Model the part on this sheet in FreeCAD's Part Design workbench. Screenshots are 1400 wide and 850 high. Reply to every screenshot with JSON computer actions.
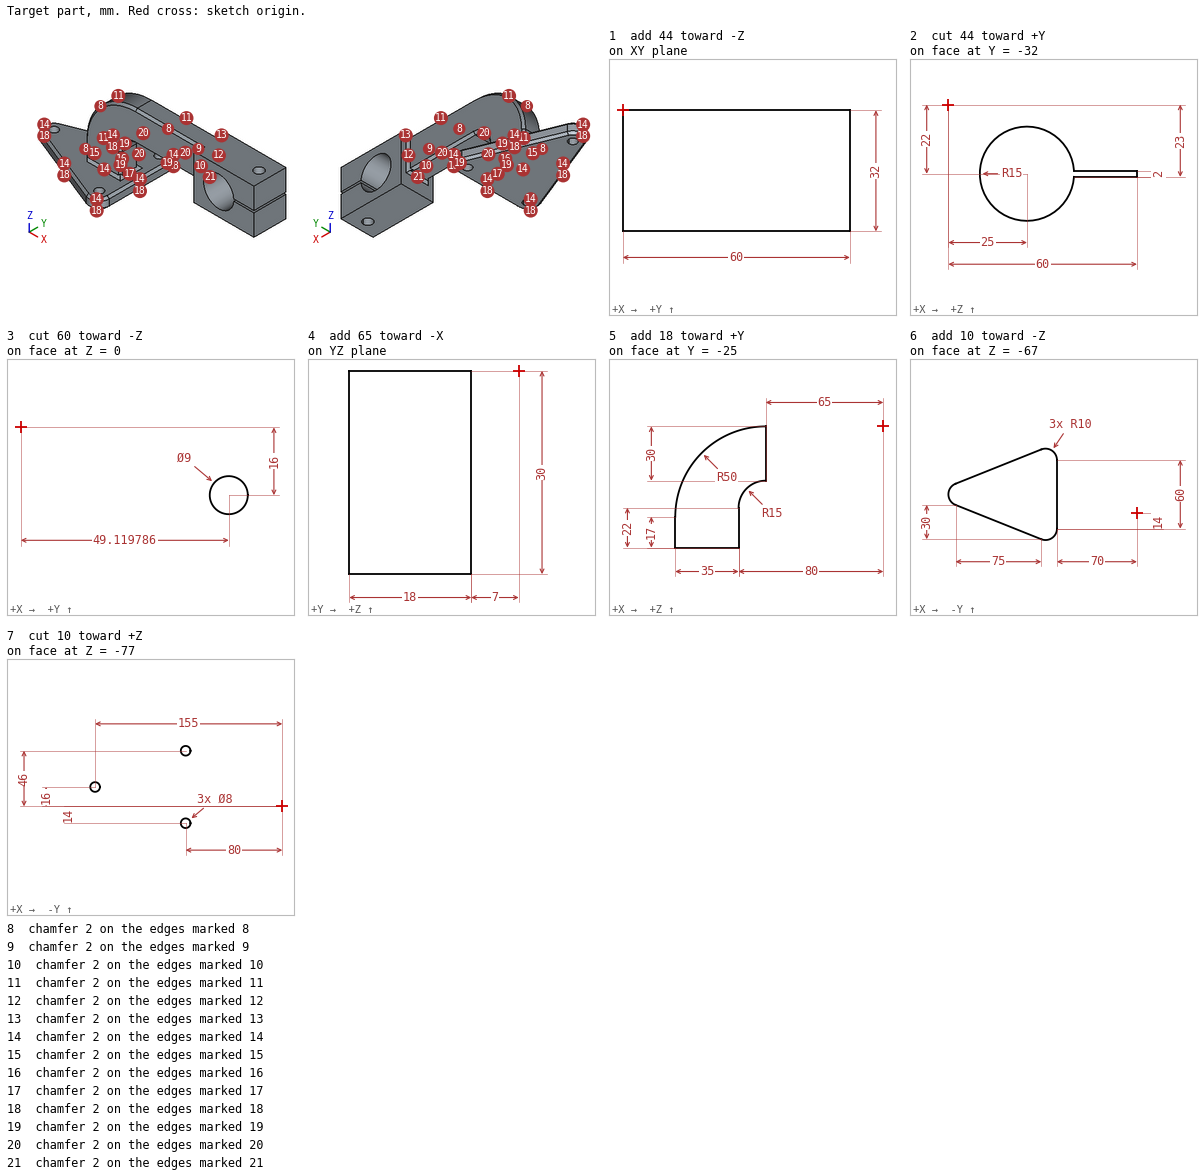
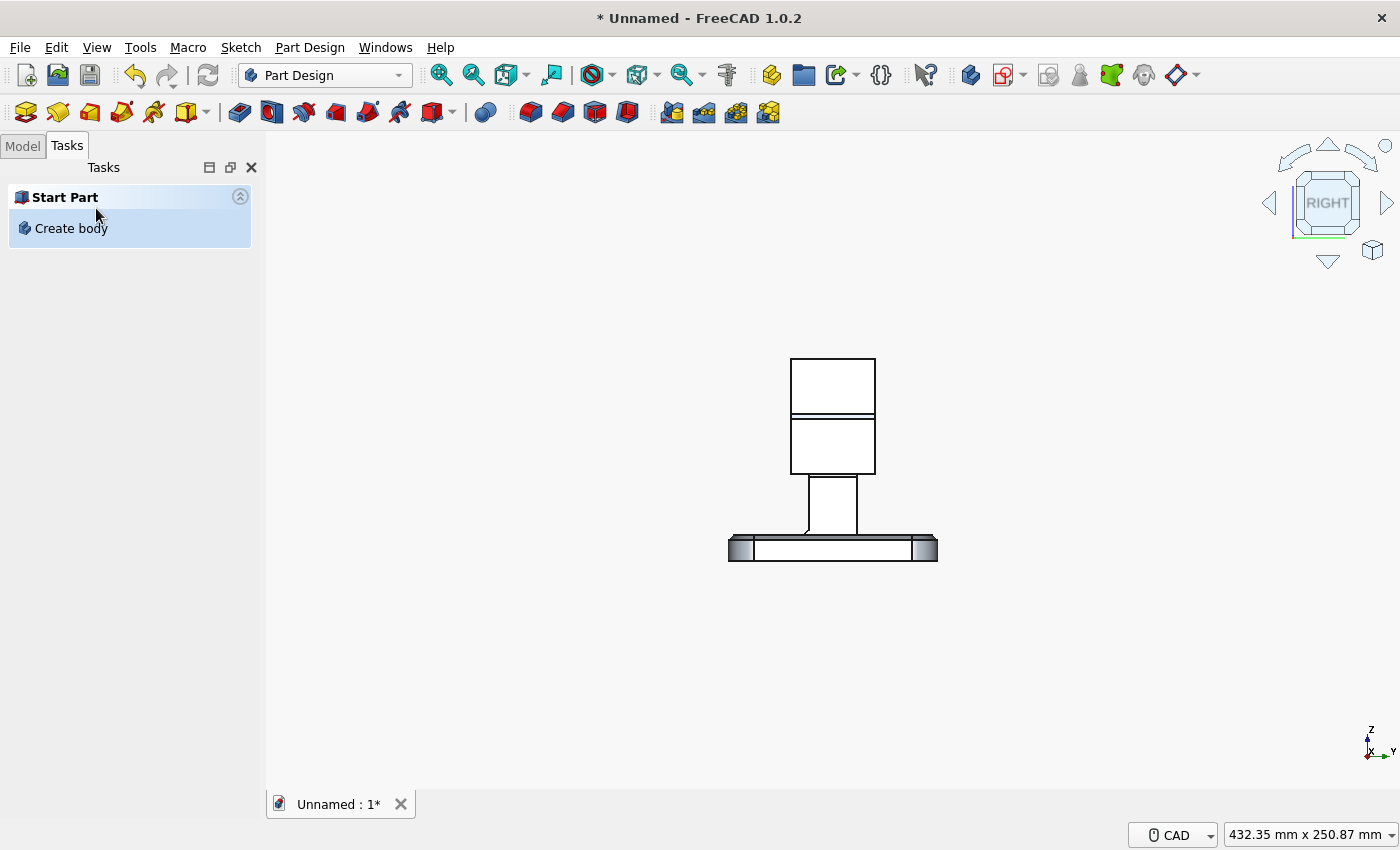
{"action": "key", "text": "5"}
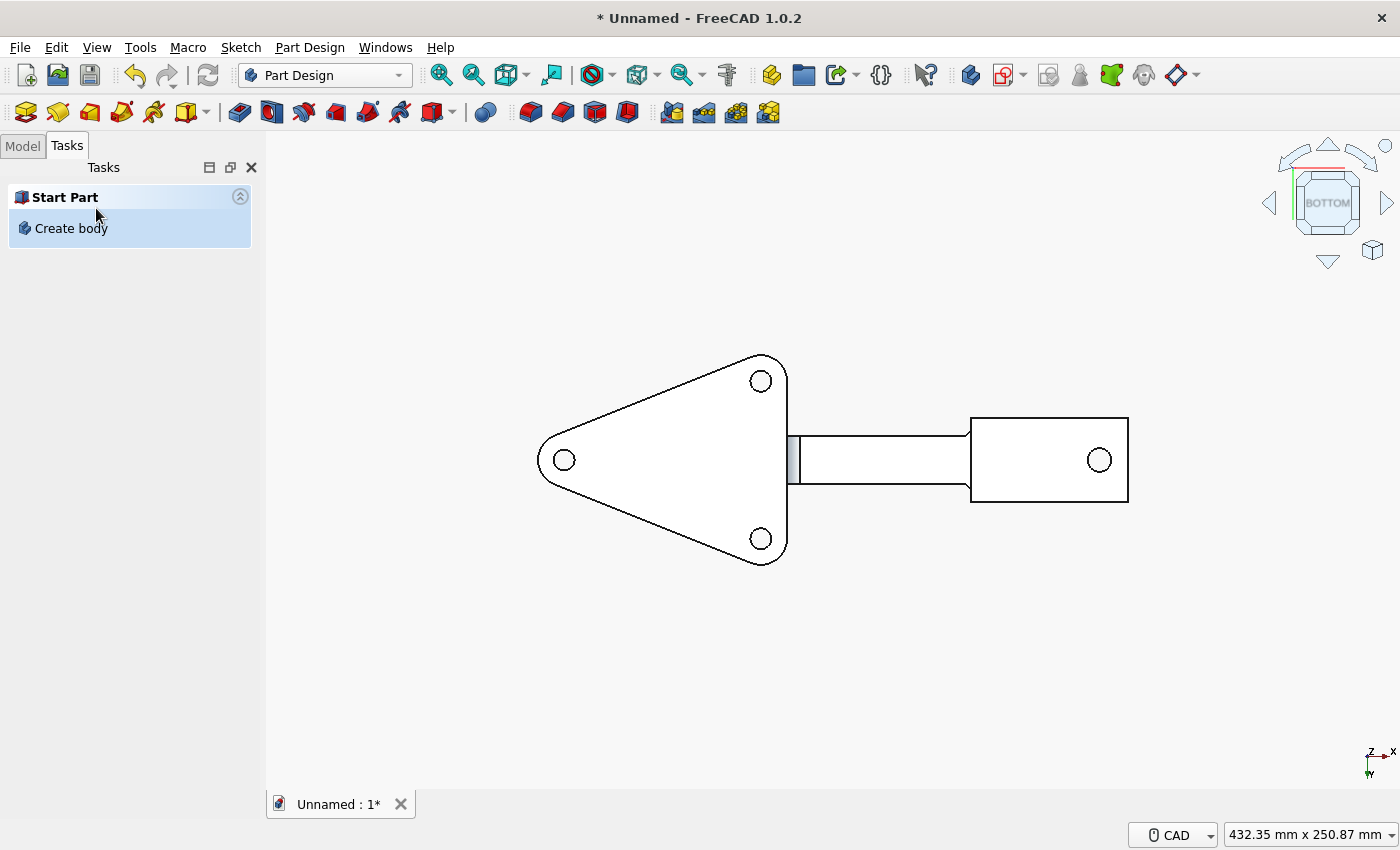
{"action": "key", "text": "4"}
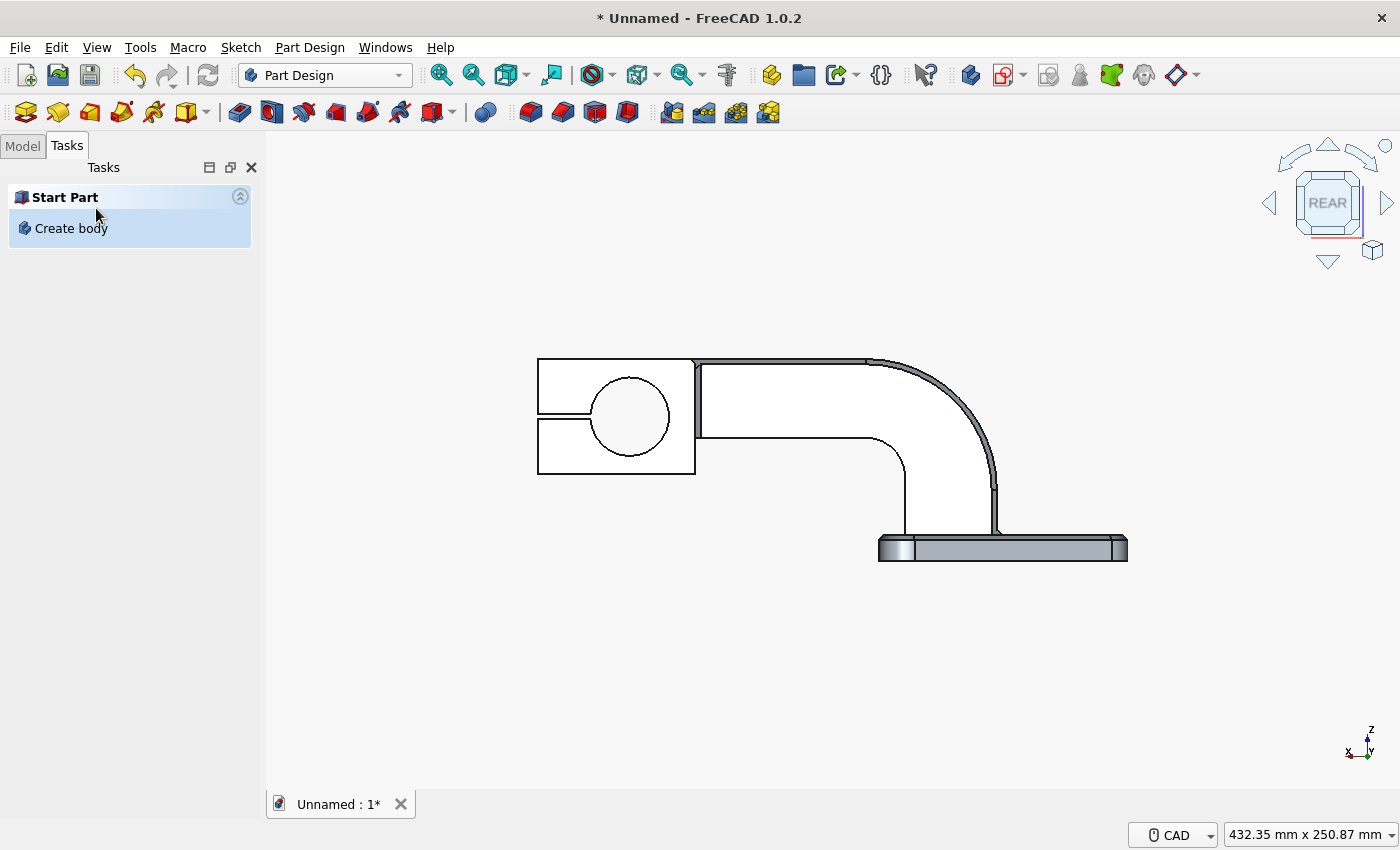
{"action": "key", "text": "6"}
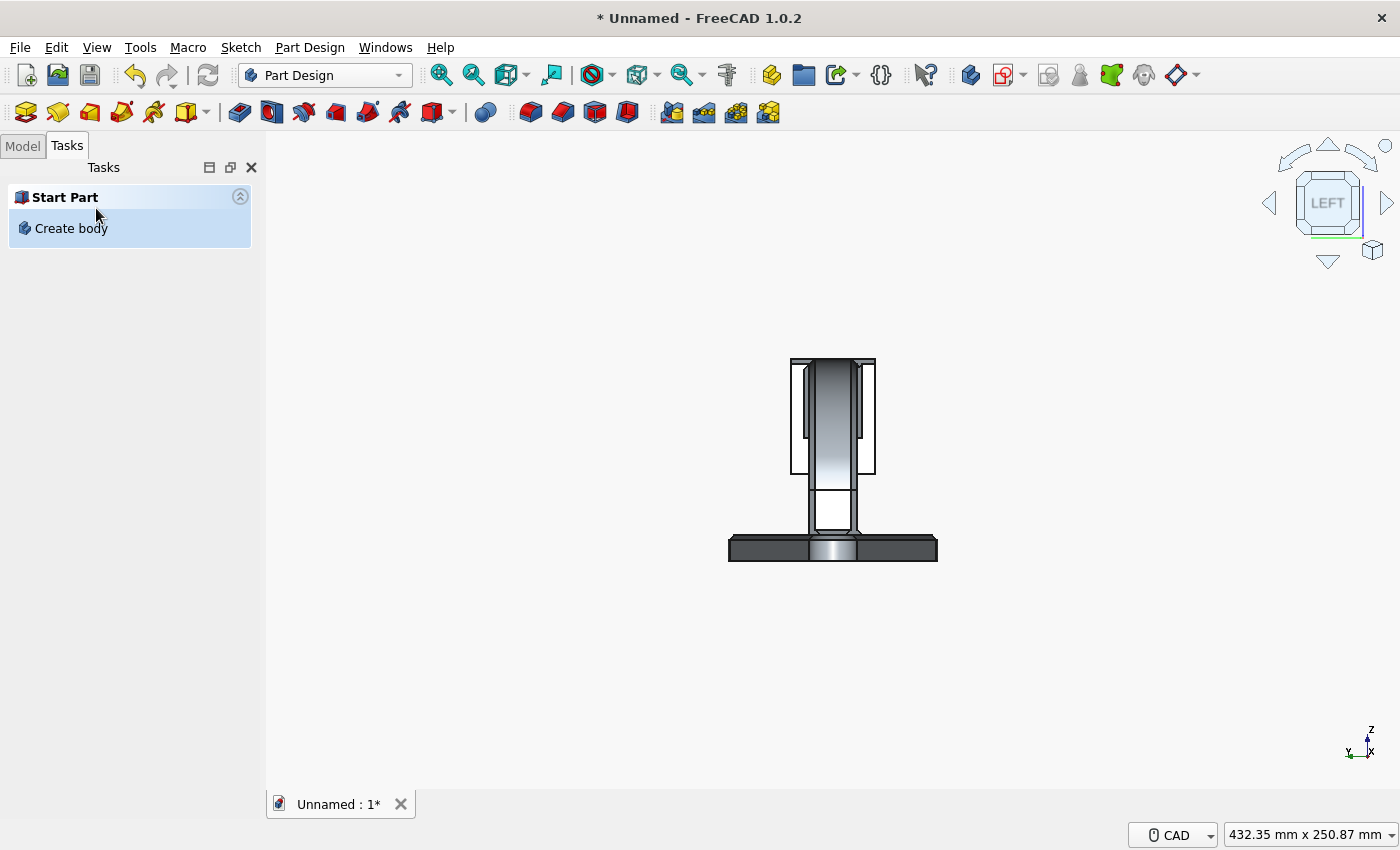
{"action": "left_click", "coordinate": [442, 76]}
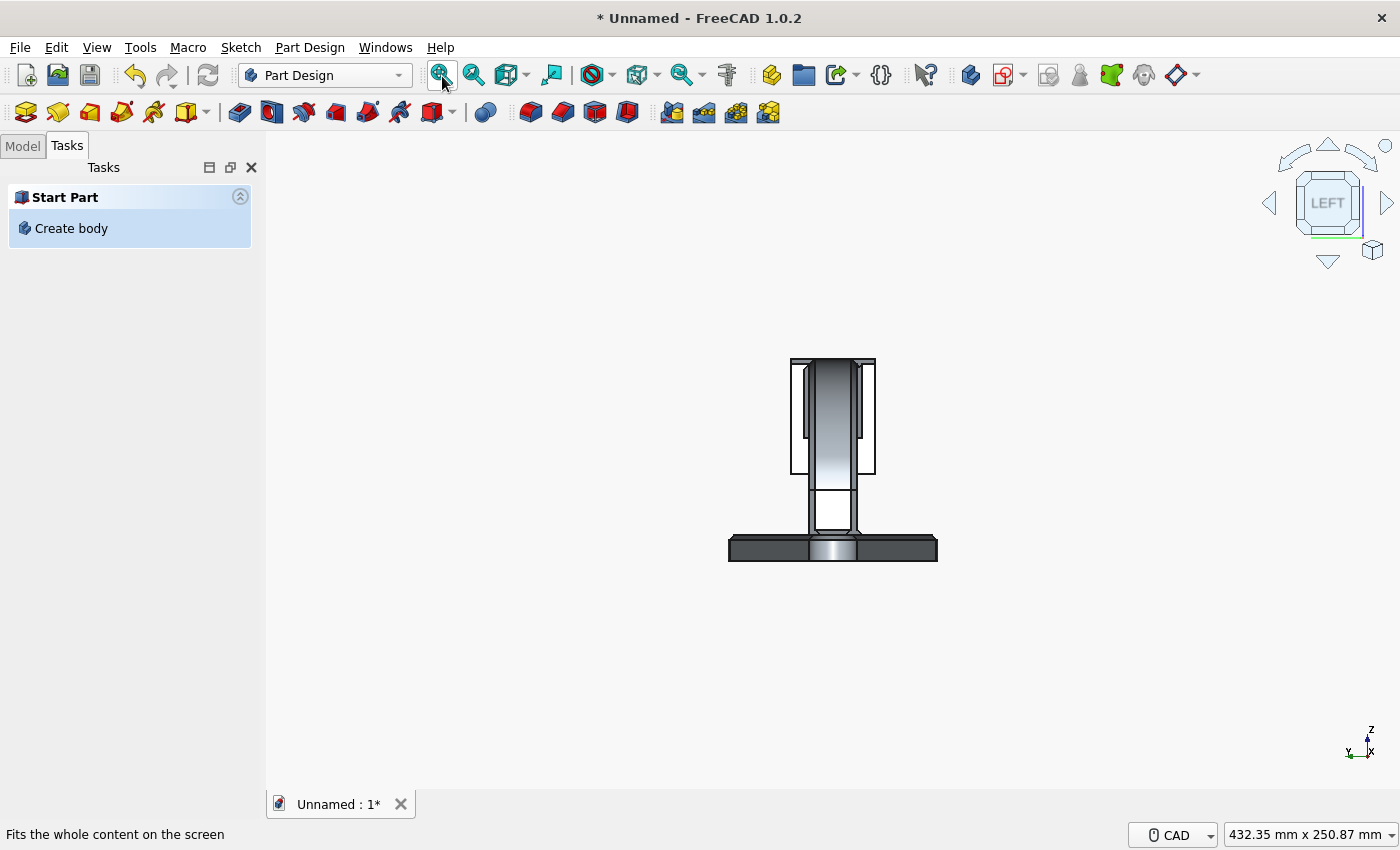
{"action": "key", "text": "v 3"}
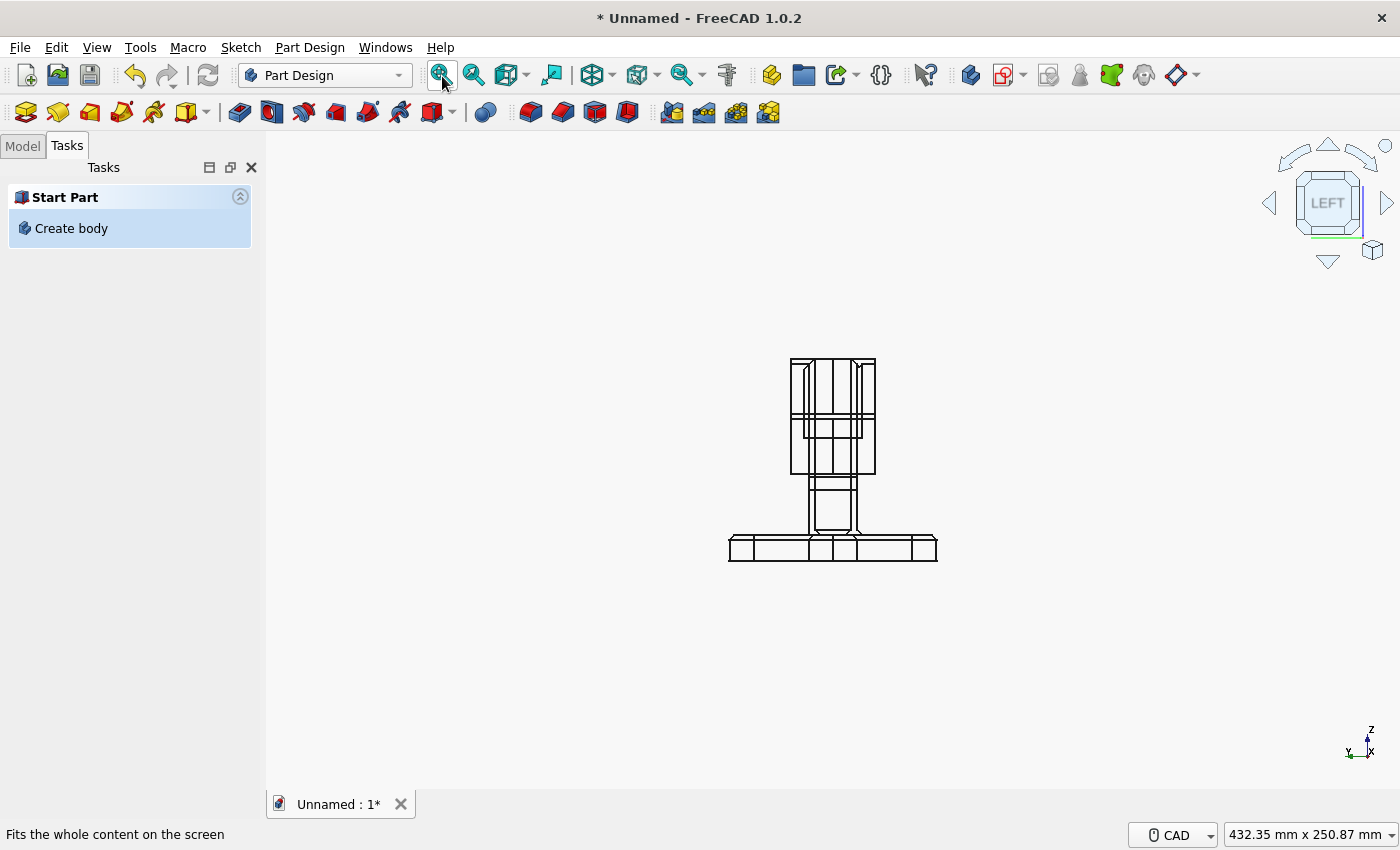
{"action": "key", "text": "0"}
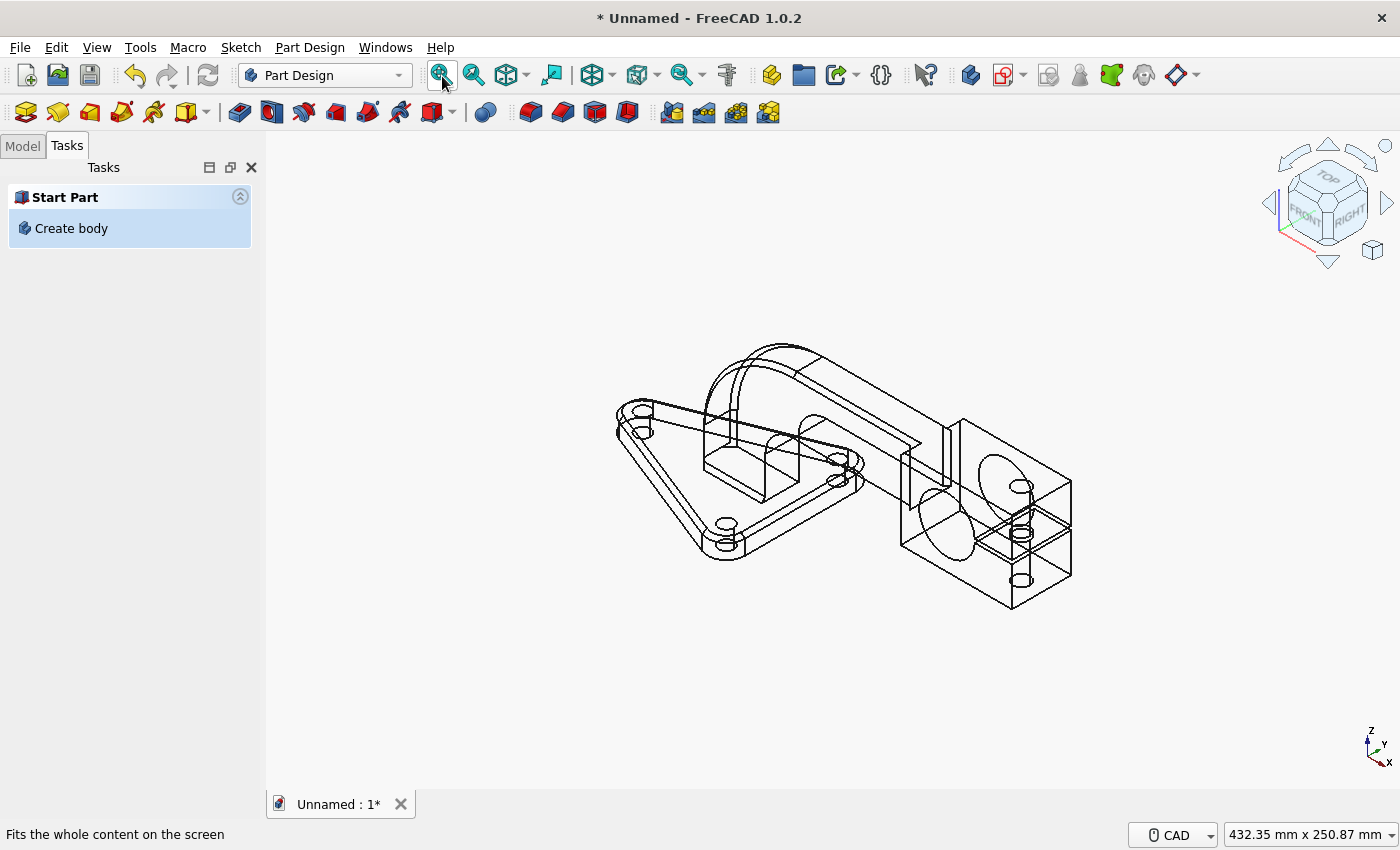
{"action": "left_click", "coordinate": [774, 467]}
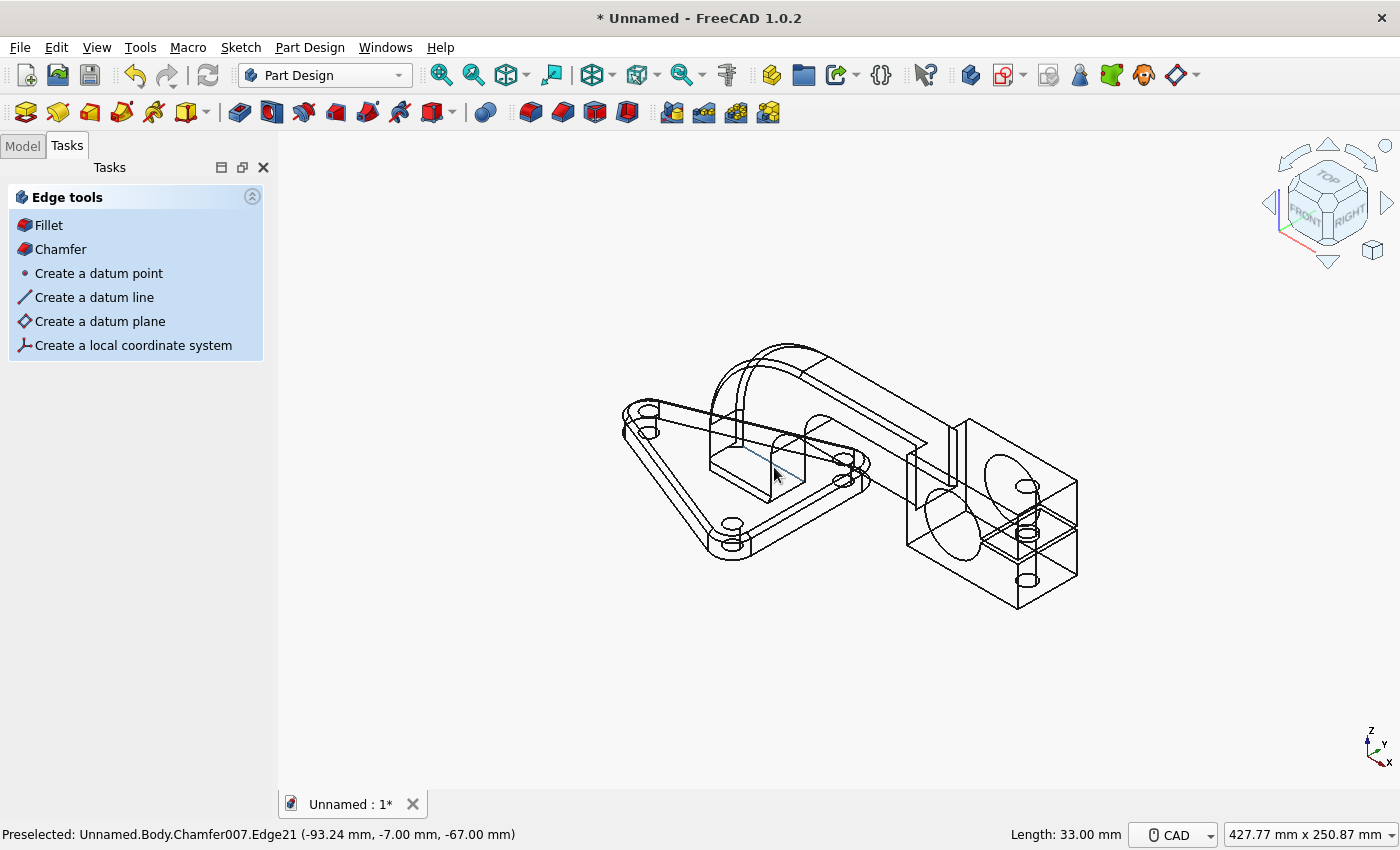
{"action": "key", "text": "v 1"}